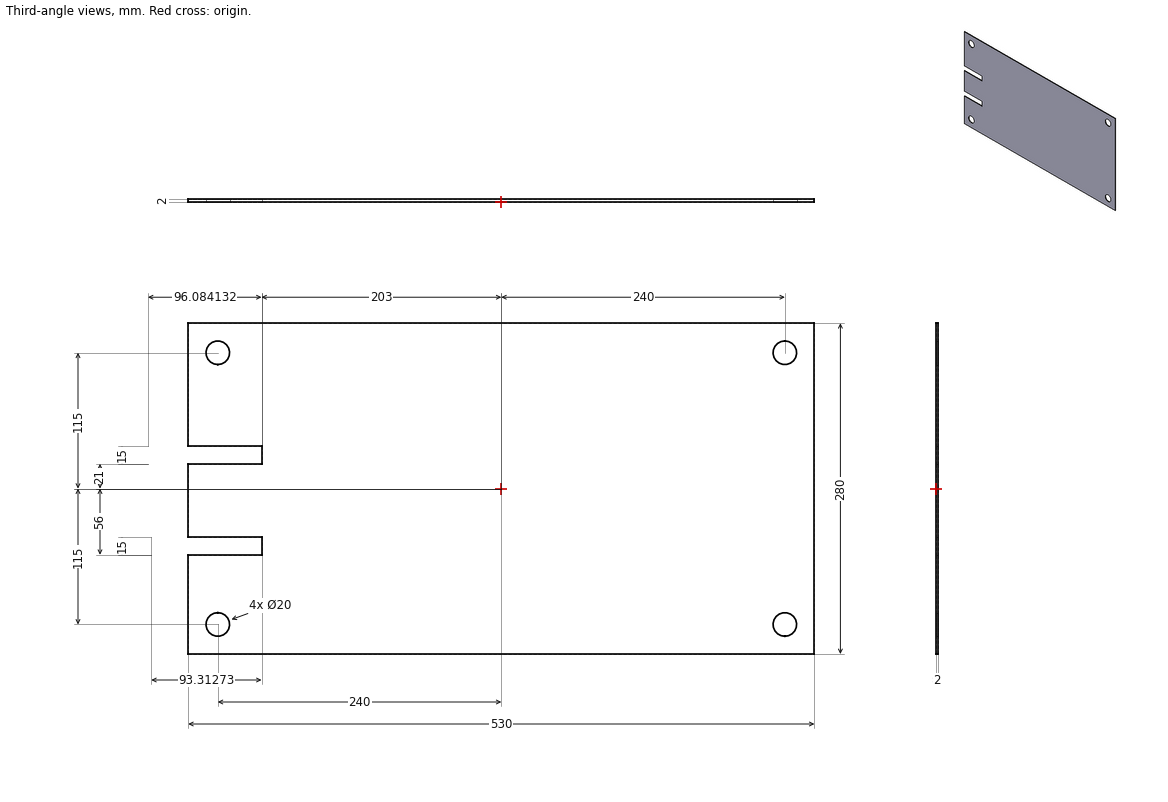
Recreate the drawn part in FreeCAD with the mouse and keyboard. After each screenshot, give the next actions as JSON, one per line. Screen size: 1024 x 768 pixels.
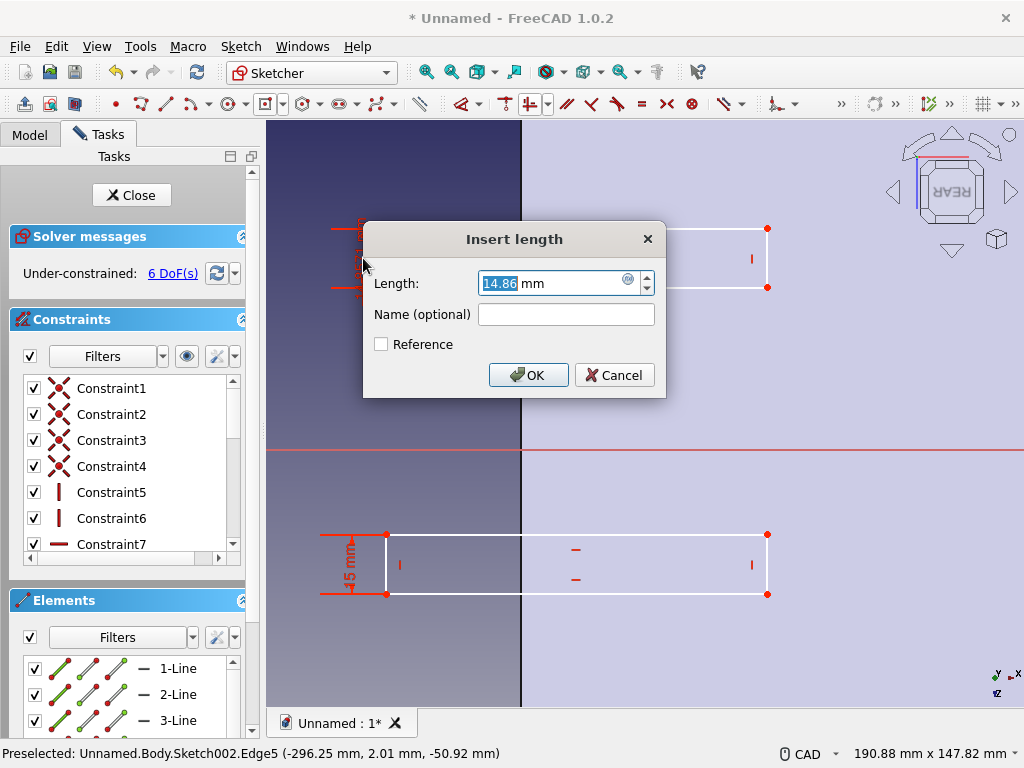
{"action": "type", "text": "15"}
{"action": "key", "text": "Return"}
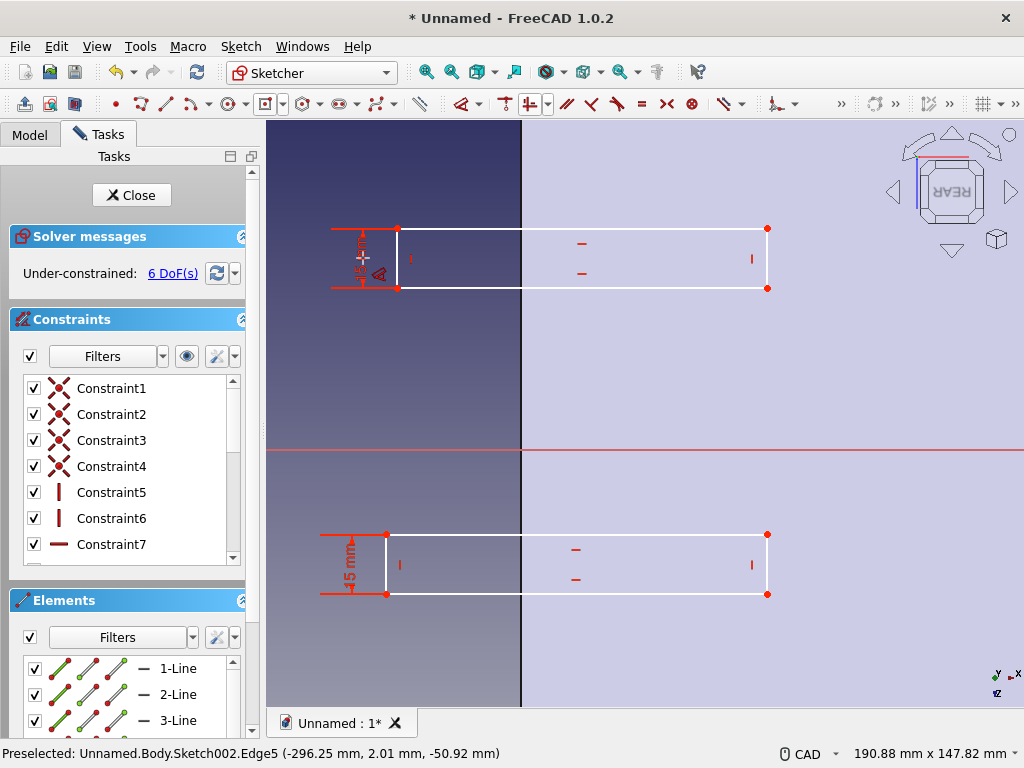
{"action": "left_click", "coordinate": [386, 535]}
{"action": "left_click", "coordinate": [352, 492]}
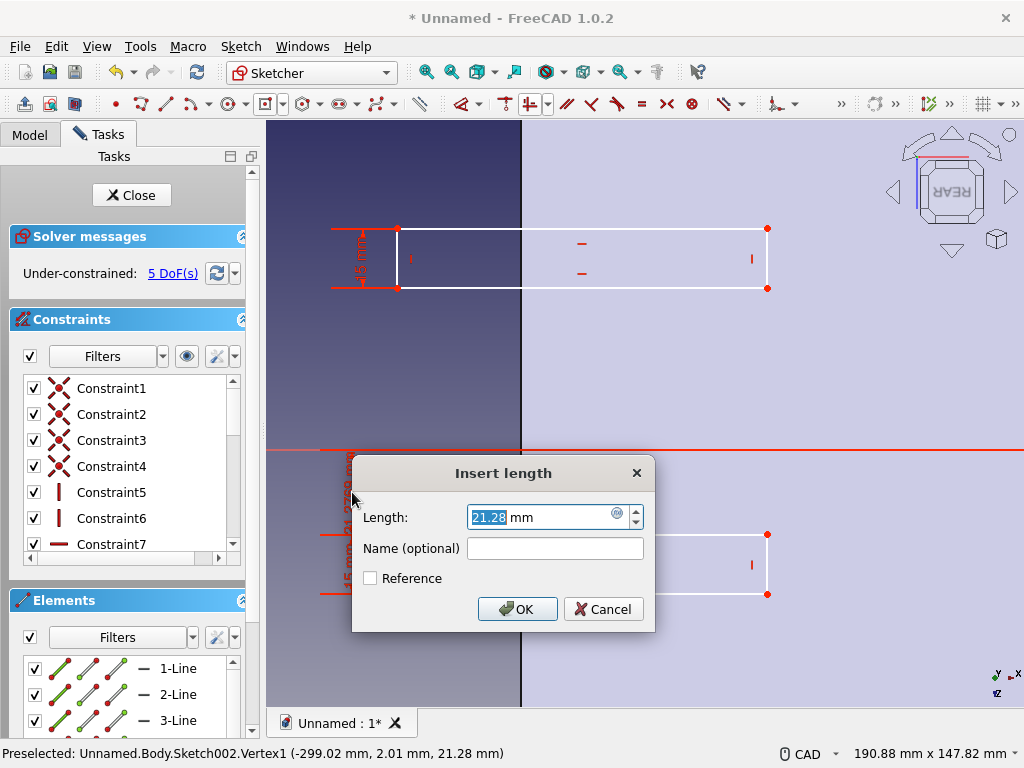
{"action": "type", "text": "21"}
{"action": "key", "text": "Return"}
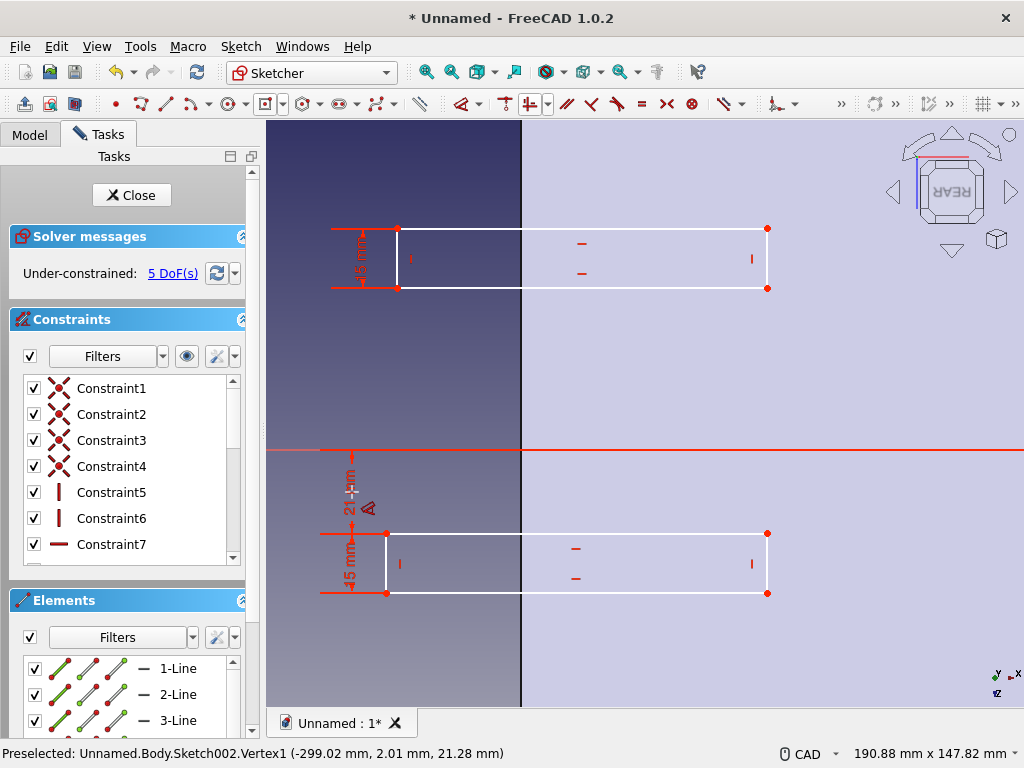
{"action": "left_click", "coordinate": [397, 229]}
{"action": "left_click", "coordinate": [363, 339]}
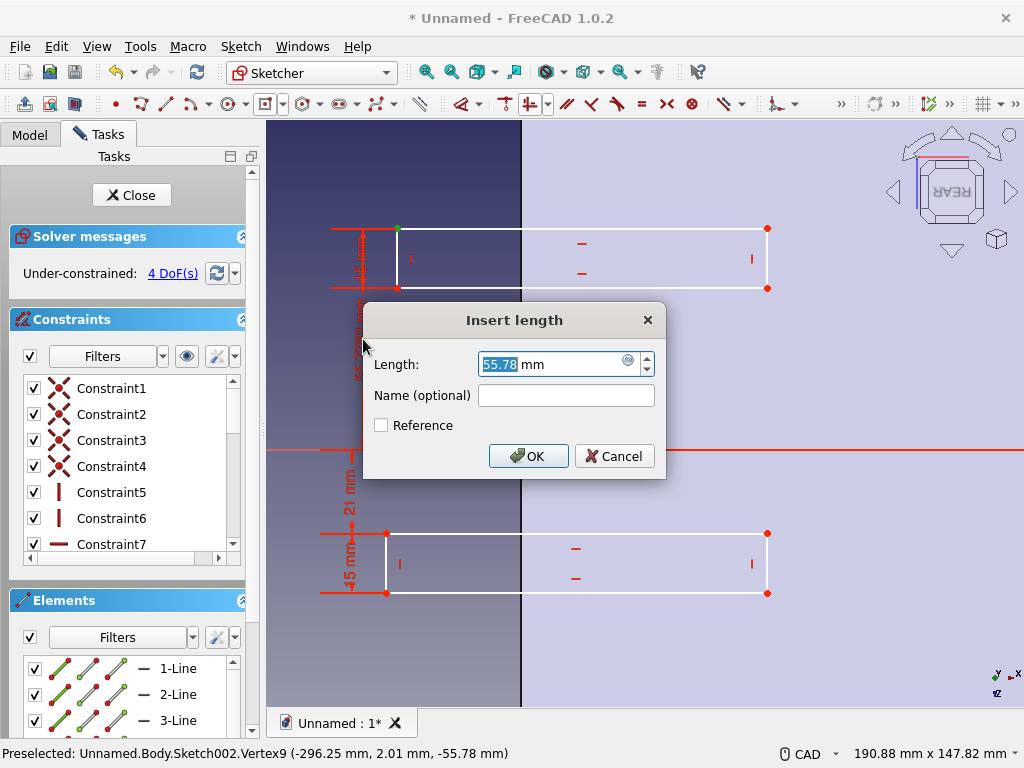
{"action": "type", "text": "56"}
{"action": "key", "text": "Return"}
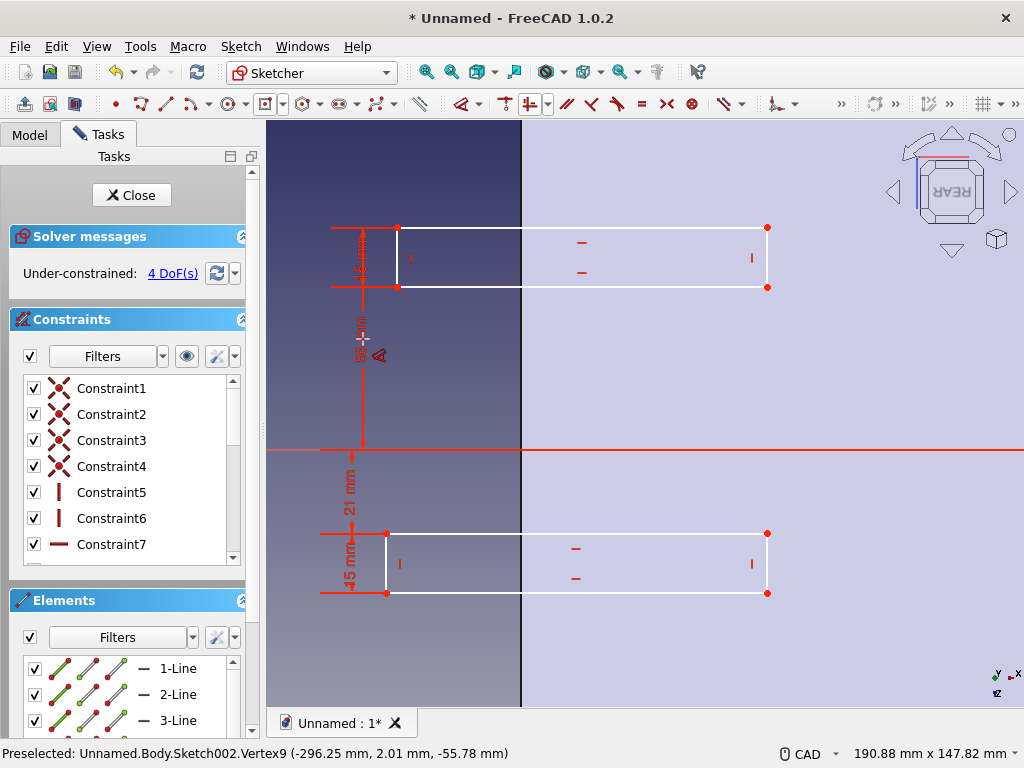
{"action": "left_click", "coordinate": [767, 593]}
{"action": "left_click", "coordinate": [813, 627]}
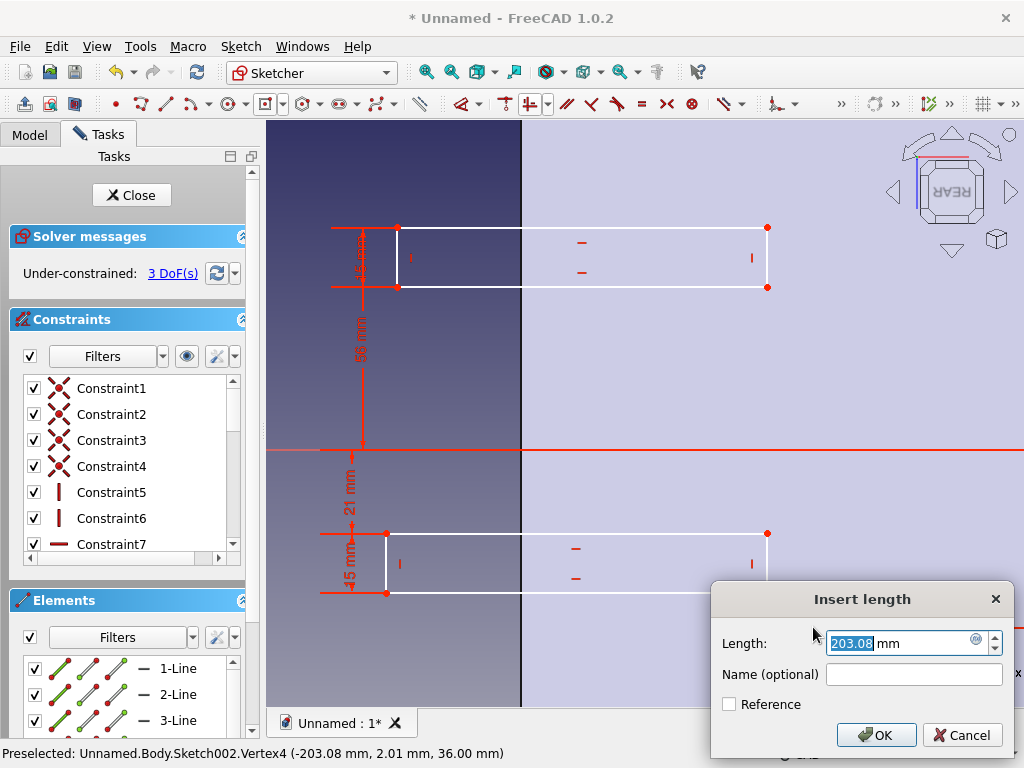
{"action": "type", "text": "203"}
{"action": "key", "text": "Return"}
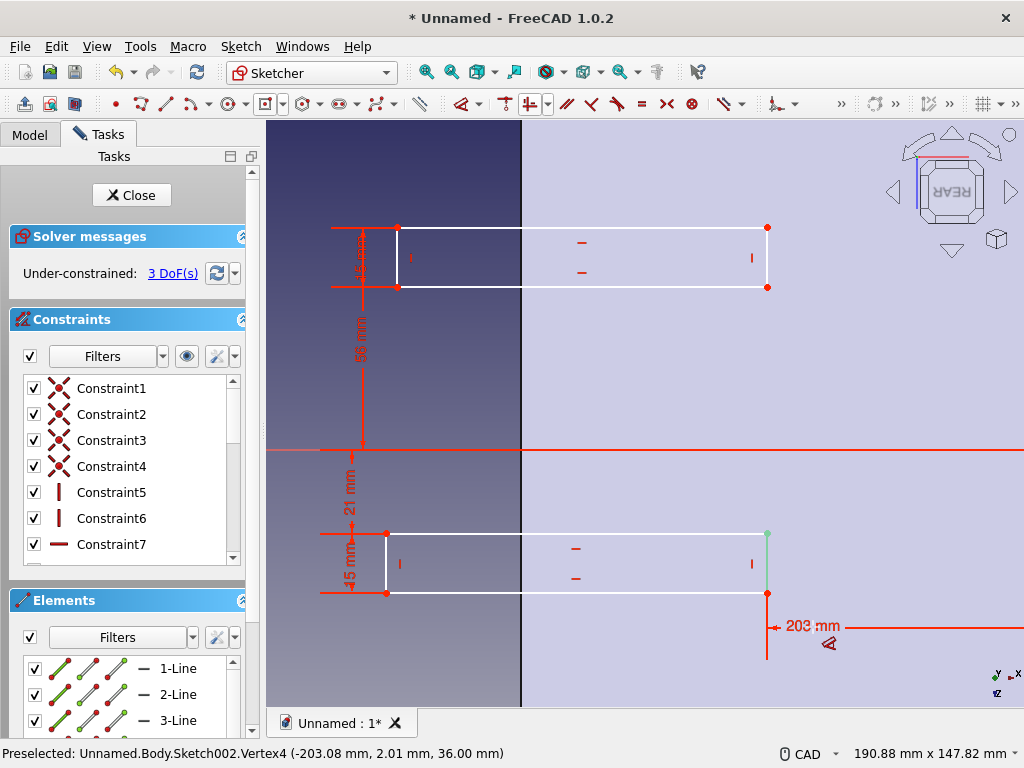
{"action": "left_click", "coordinate": [767, 287]}
{"action": "left_click", "coordinate": [813, 253]}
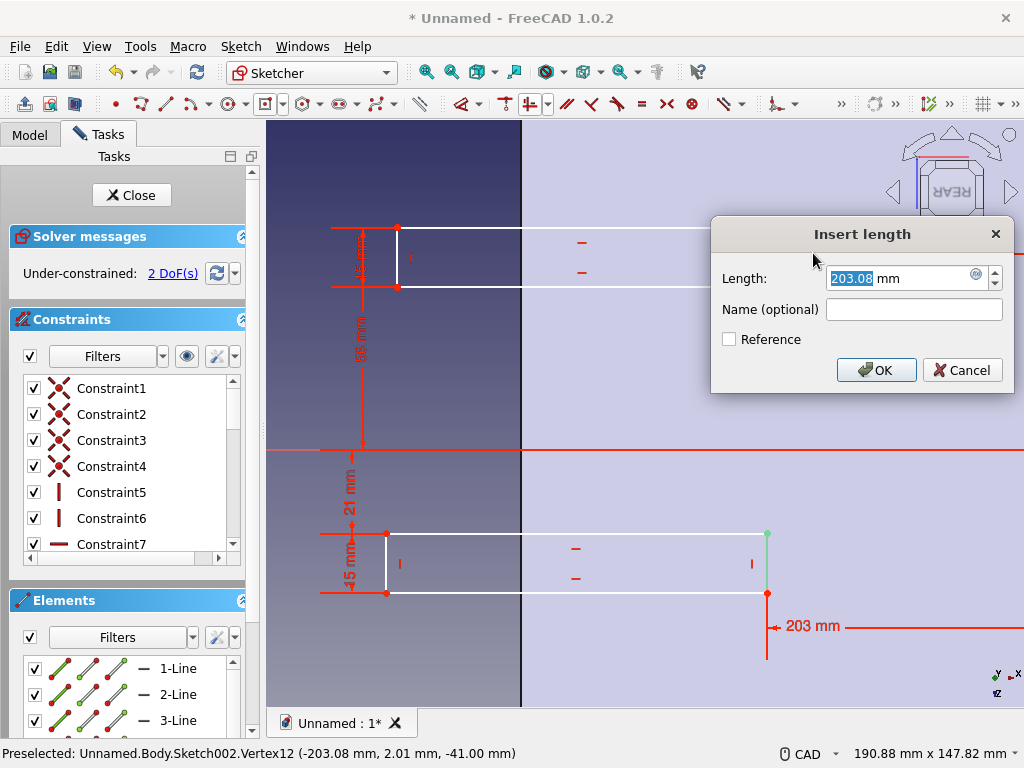
{"action": "type", "text": "203"}
{"action": "key", "text": "Return"}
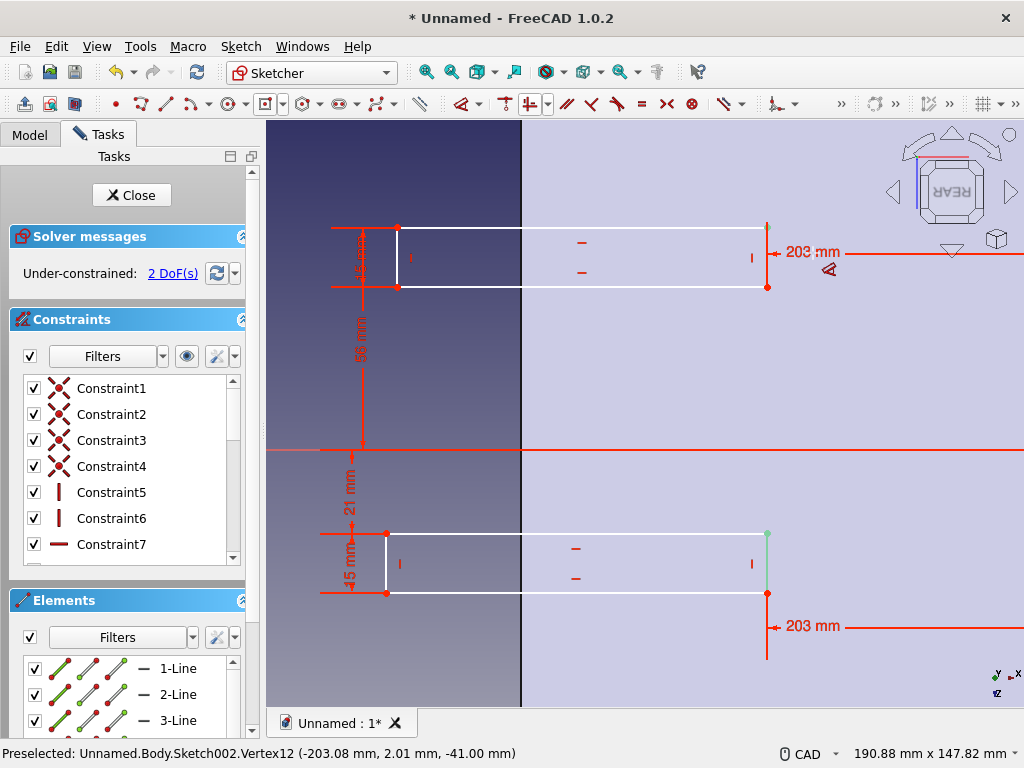
{"action": "left_click", "coordinate": [508, 287]}
{"action": "left_click", "coordinate": [582, 253]}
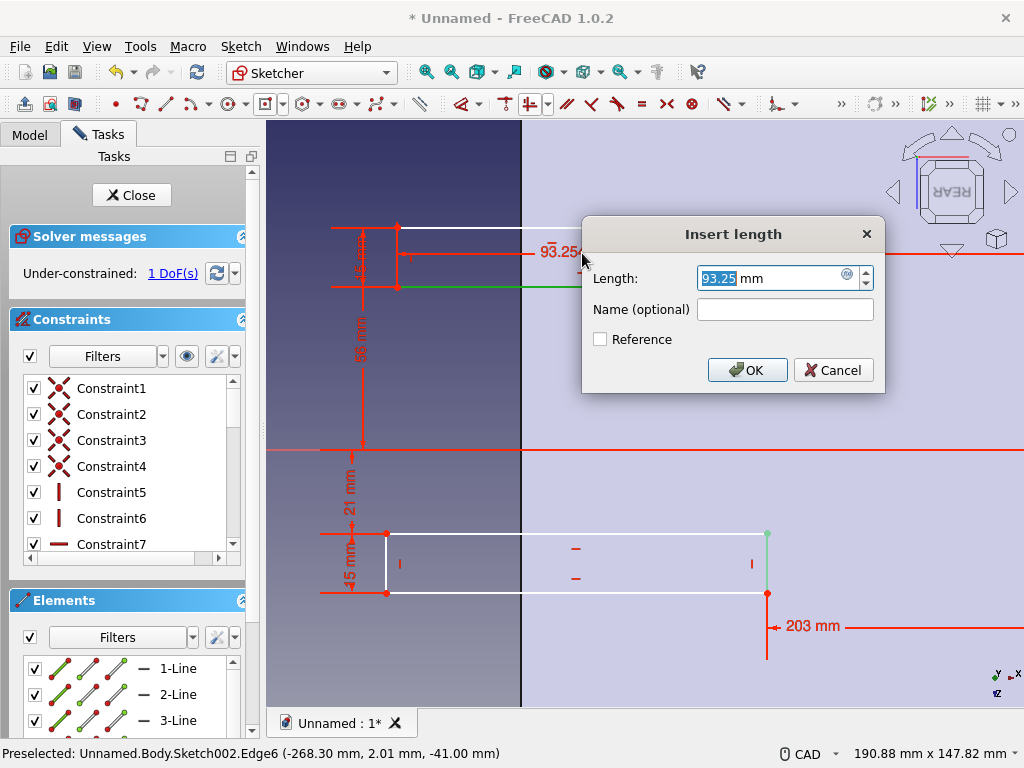
{"action": "type", "text": "93.31273"}
{"action": "key", "text": "Return"}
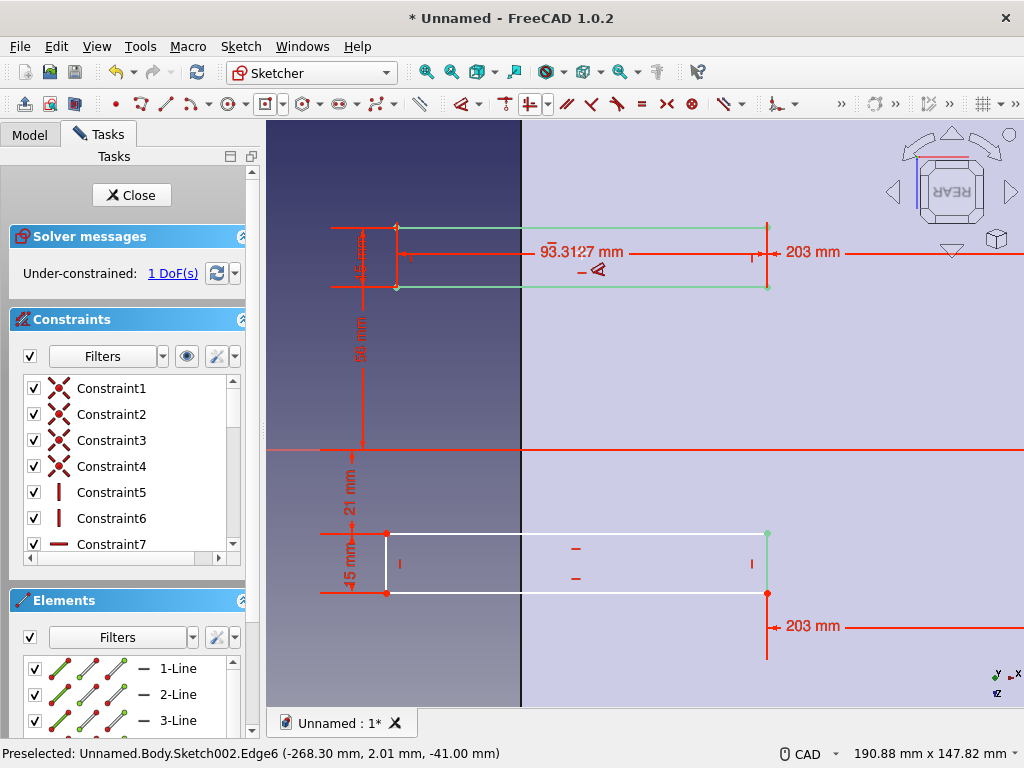
{"action": "left_click", "coordinate": [500, 593]}
{"action": "left_click", "coordinate": [577, 627]}